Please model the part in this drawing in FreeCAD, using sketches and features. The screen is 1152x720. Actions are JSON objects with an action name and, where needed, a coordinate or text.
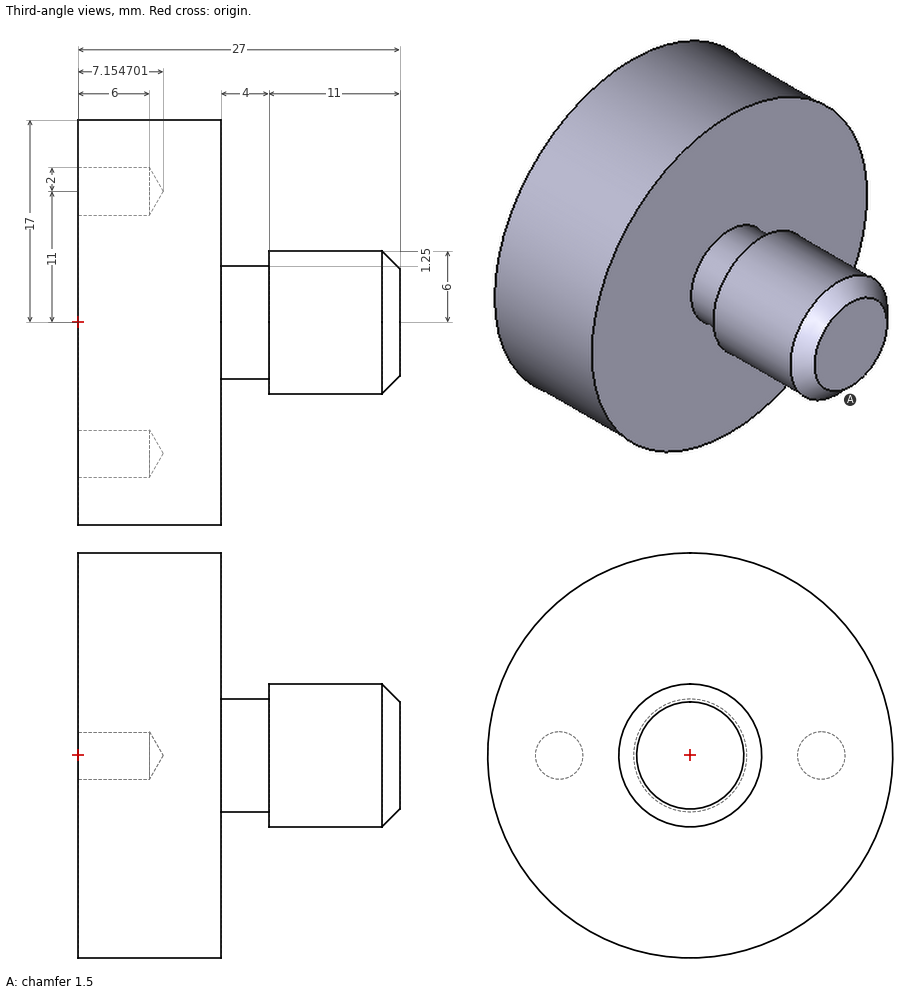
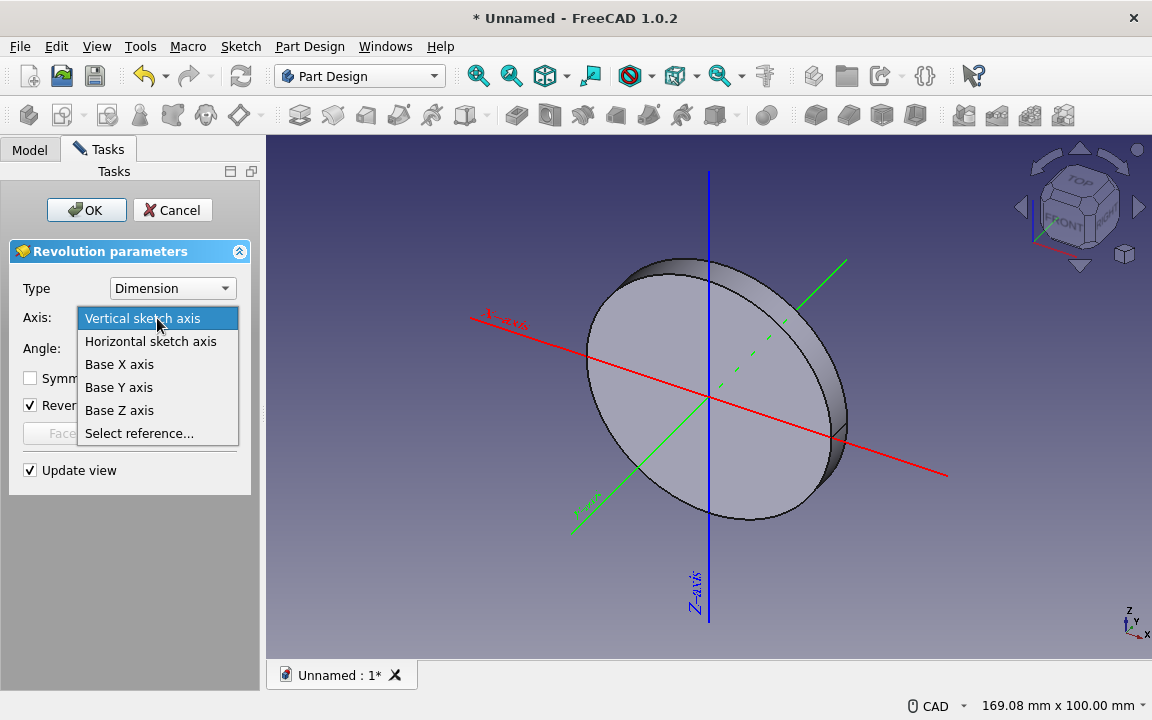
{"action": "left_click", "coordinate": [156, 342]}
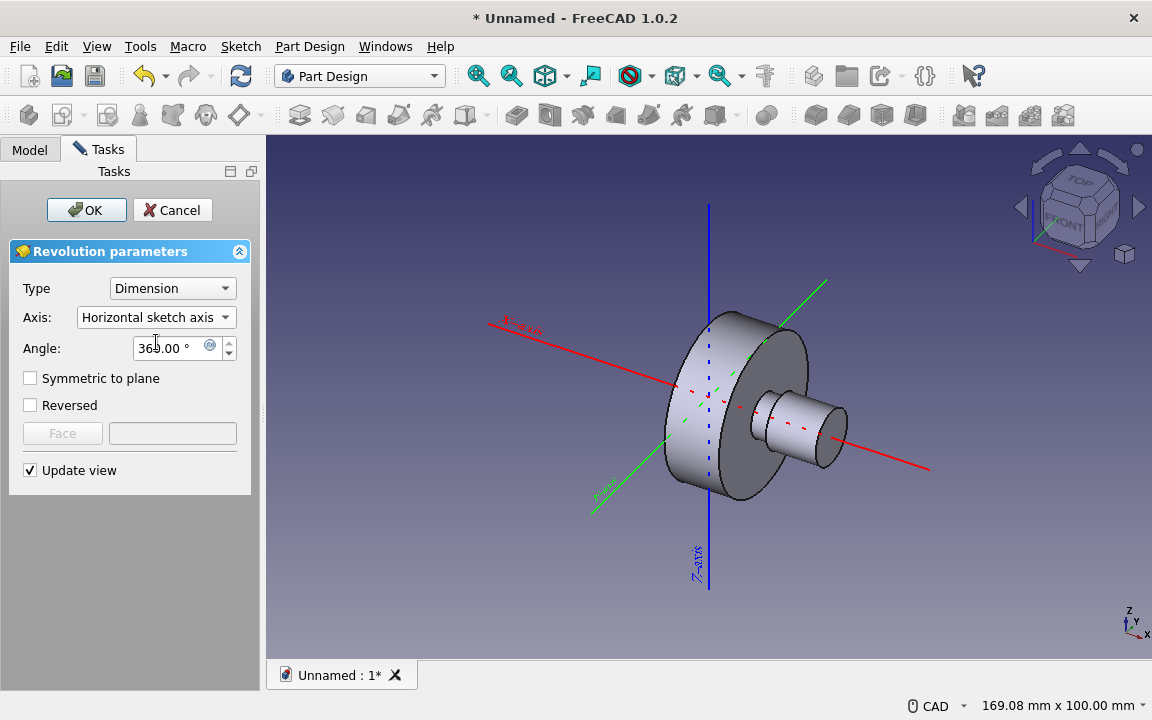
{"action": "left_click", "coordinate": [87, 210]}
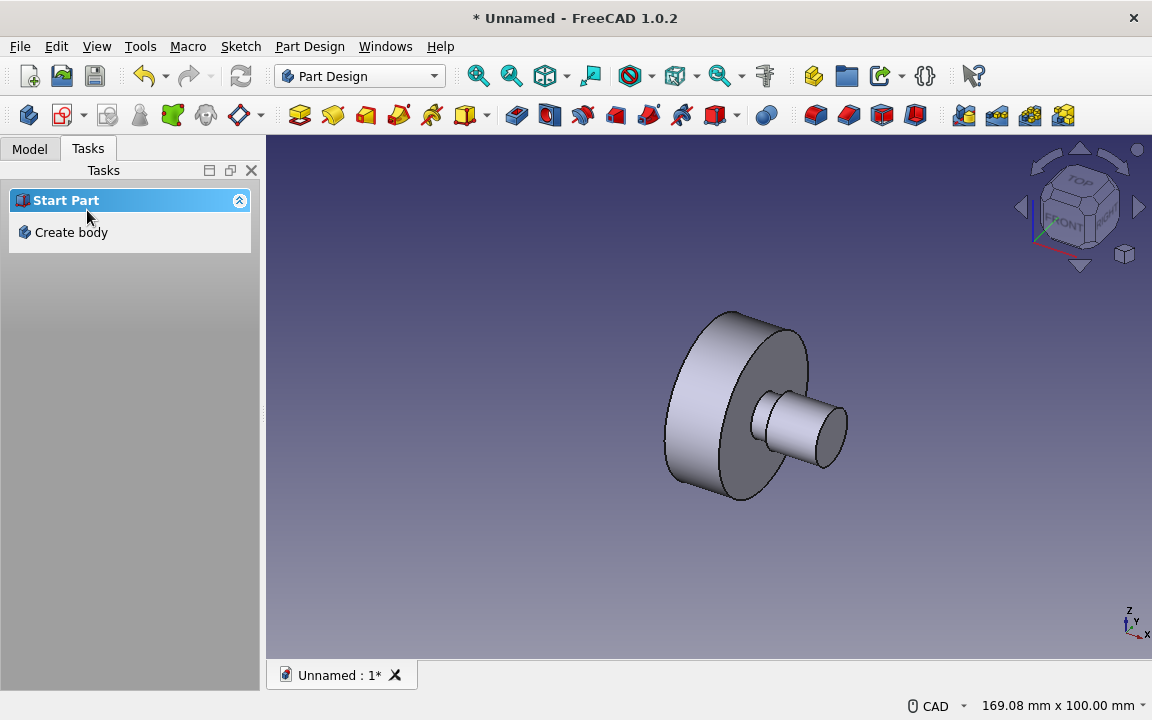
{"action": "left_click", "coordinate": [816, 452]}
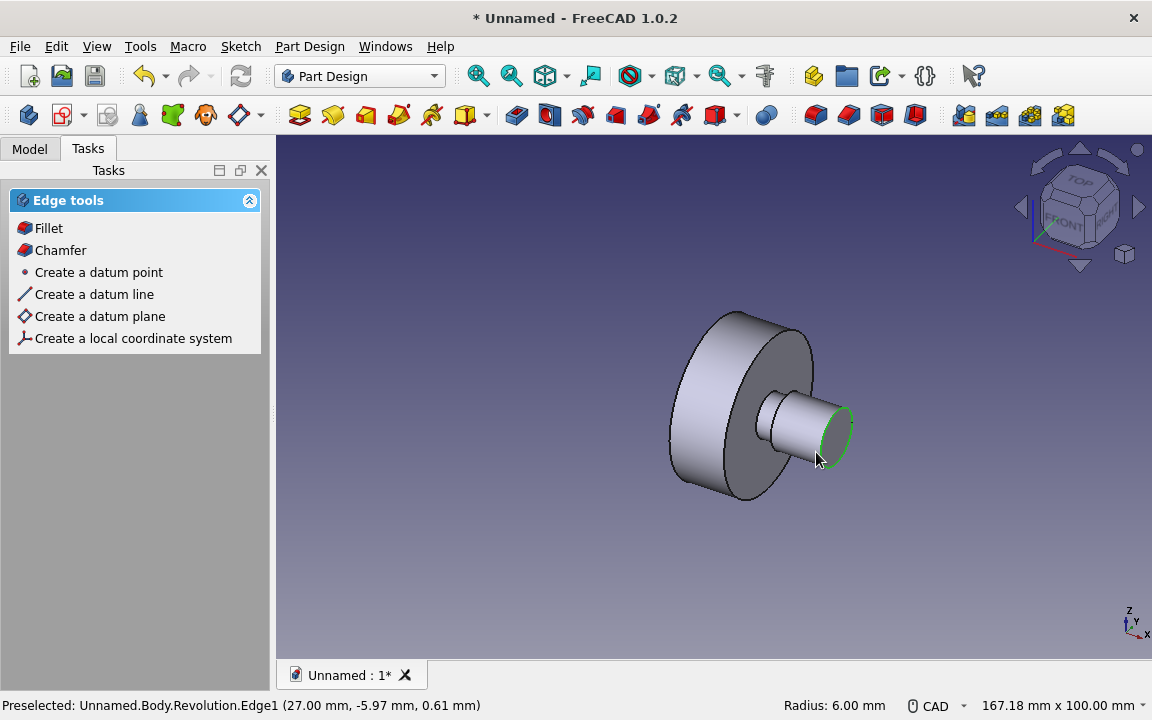
{"action": "left_click", "coordinate": [849, 116]}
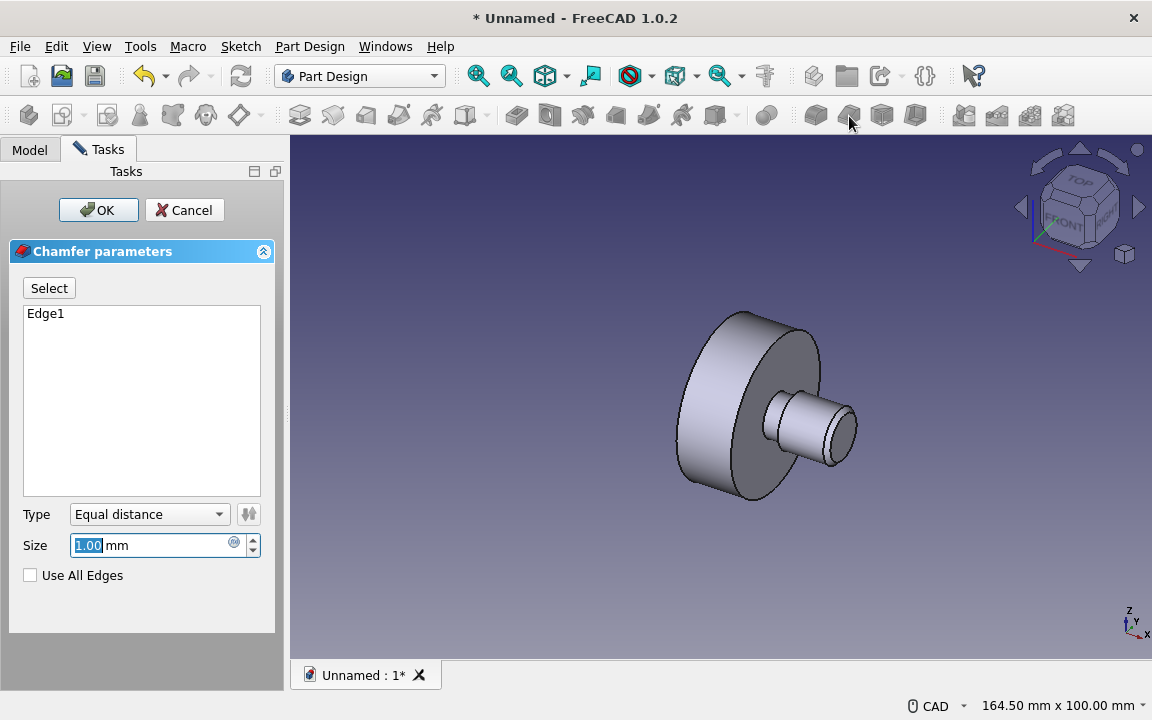
{"action": "type", "text": "1.5"}
{"action": "key", "text": "Tab"}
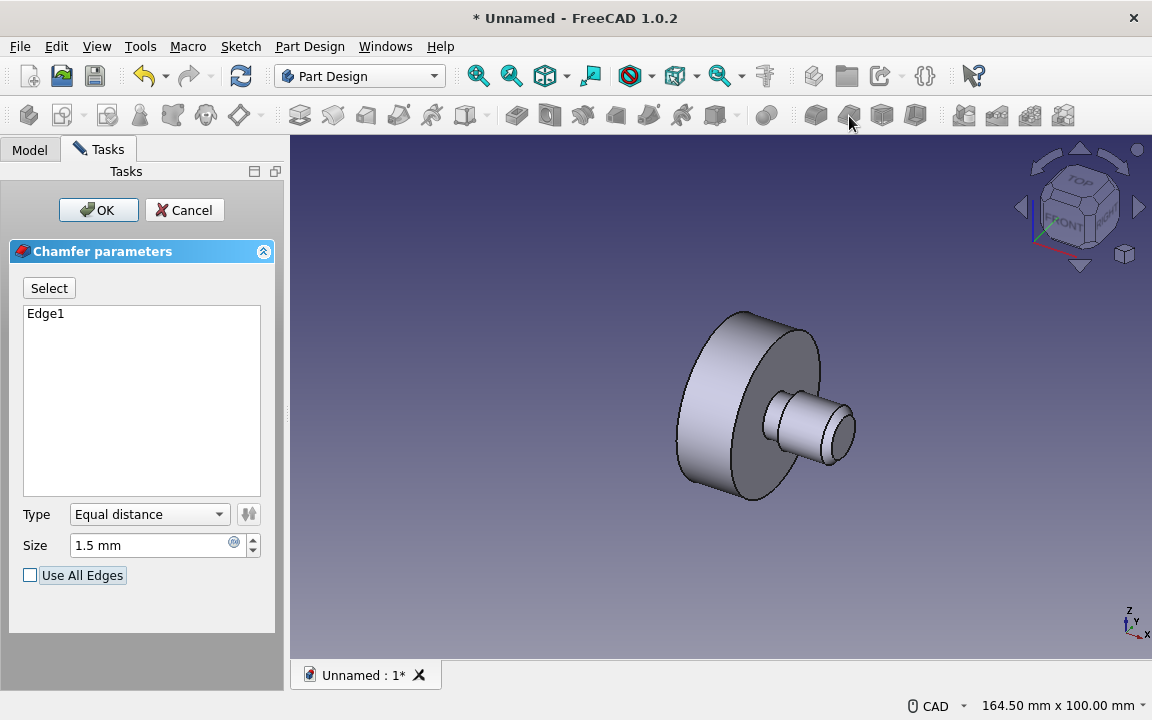
{"action": "left_click", "coordinate": [99, 210]}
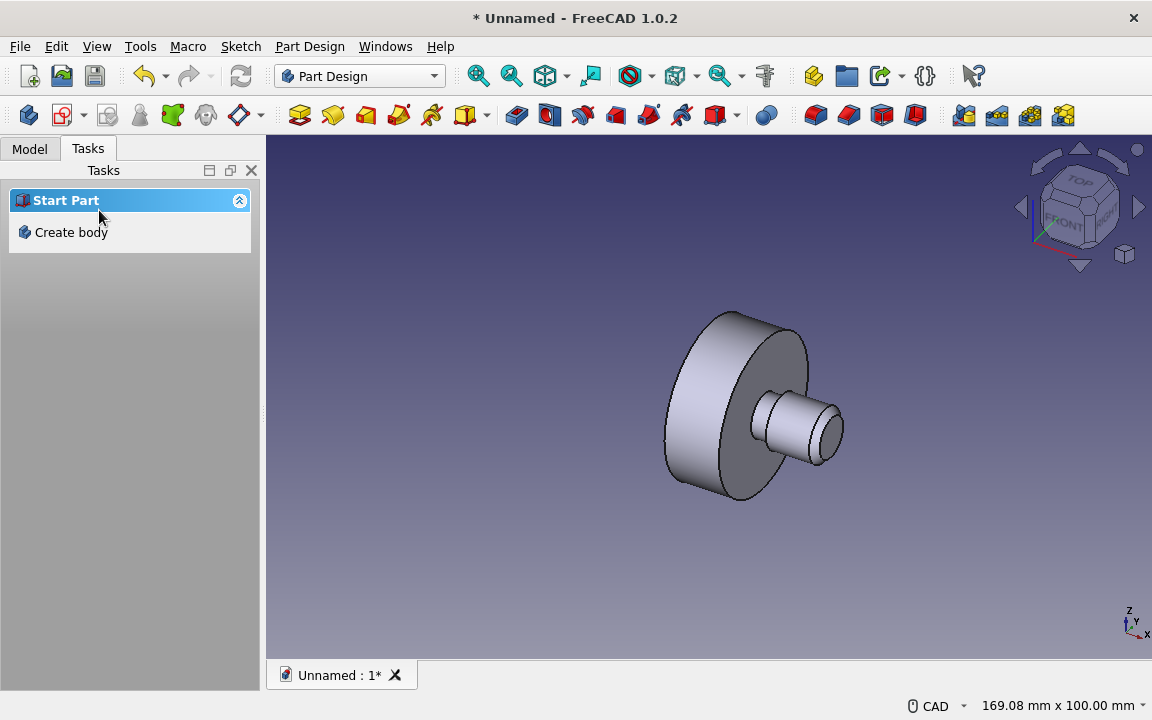
{"action": "left_click", "coordinate": [62, 116]}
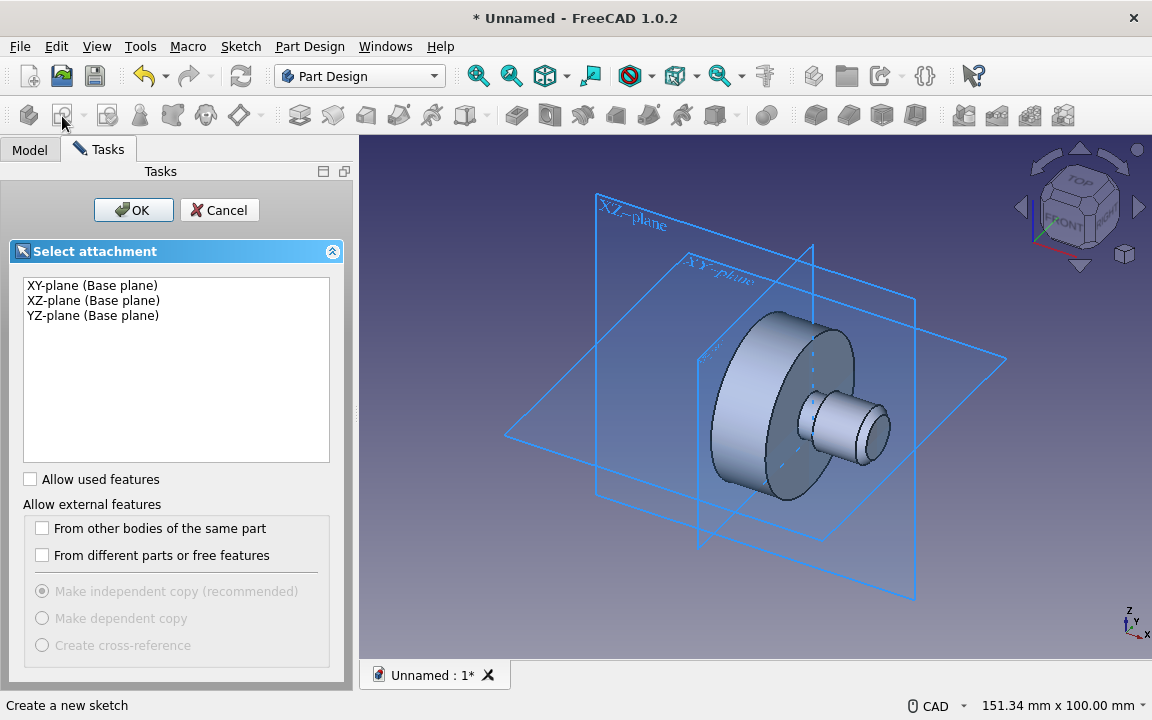
{"action": "left_click", "coordinate": [84, 286]}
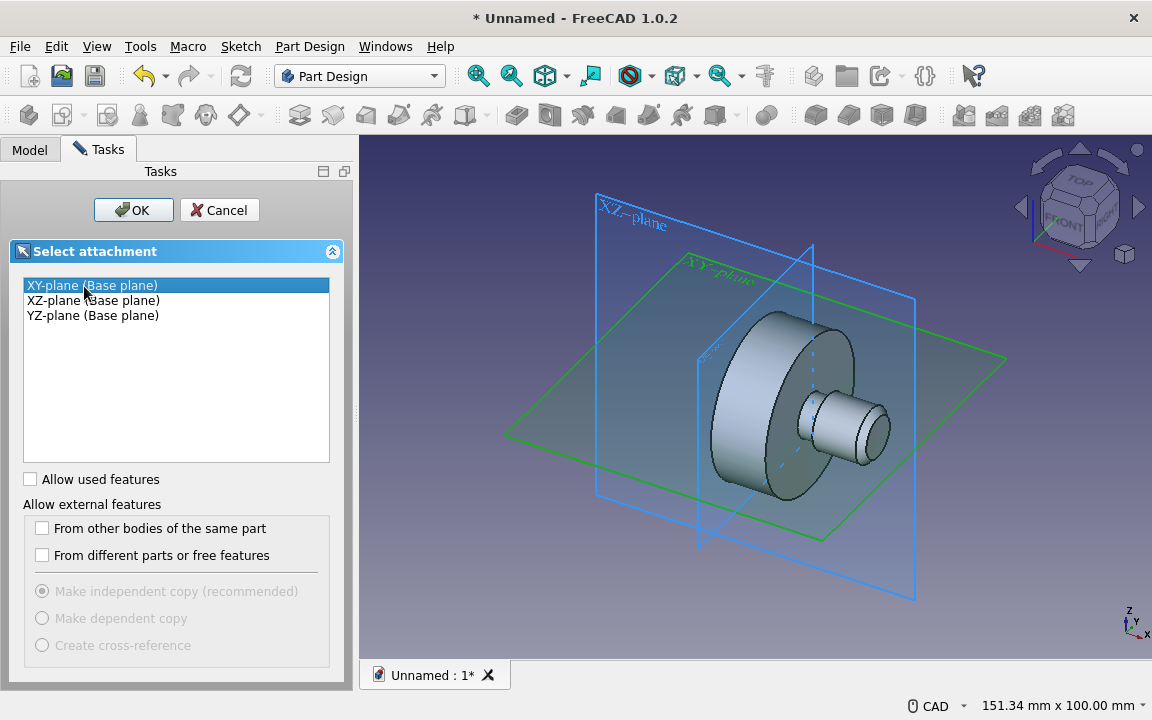
{"action": "left_click", "coordinate": [134, 210]}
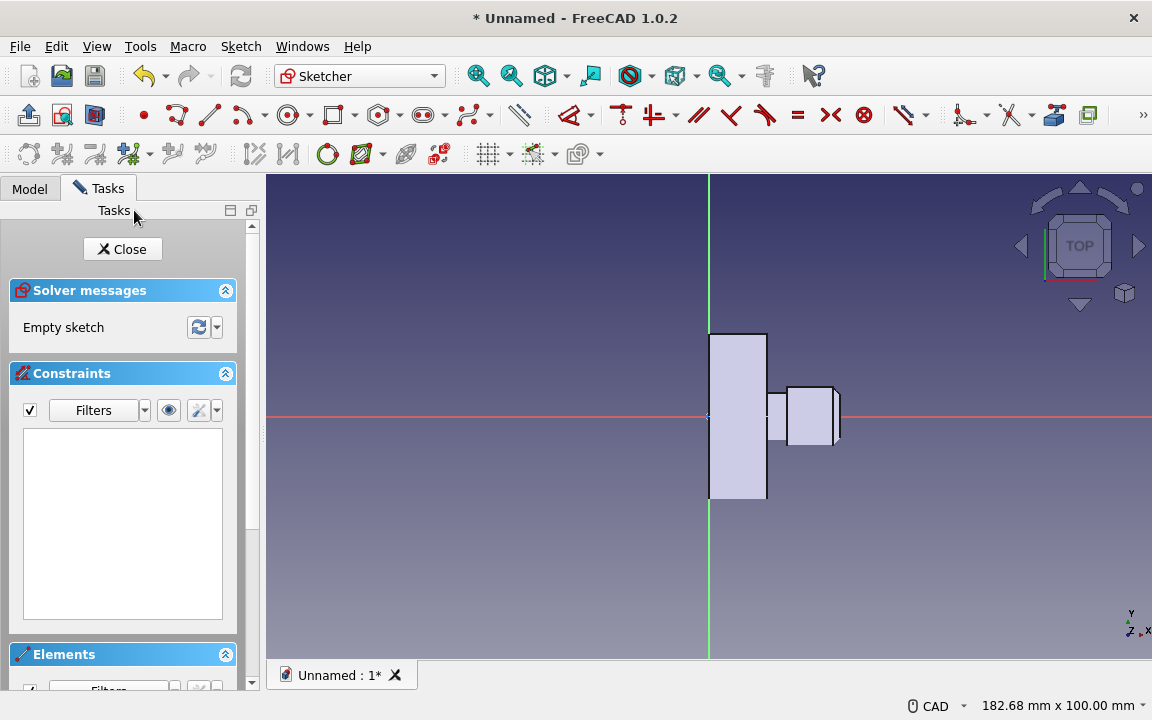
{"action": "key", "text": "q s"}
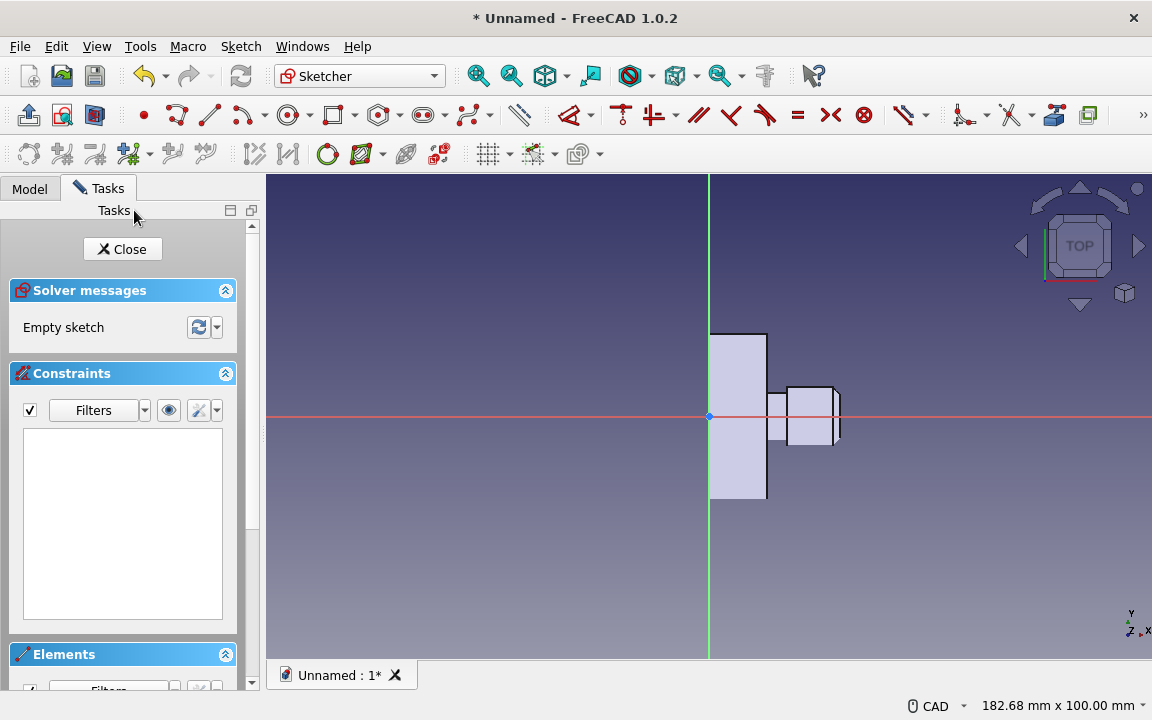
{"action": "scroll", "coordinate": [757, 377], "scroll_direction": "up", "scroll_amount": 8}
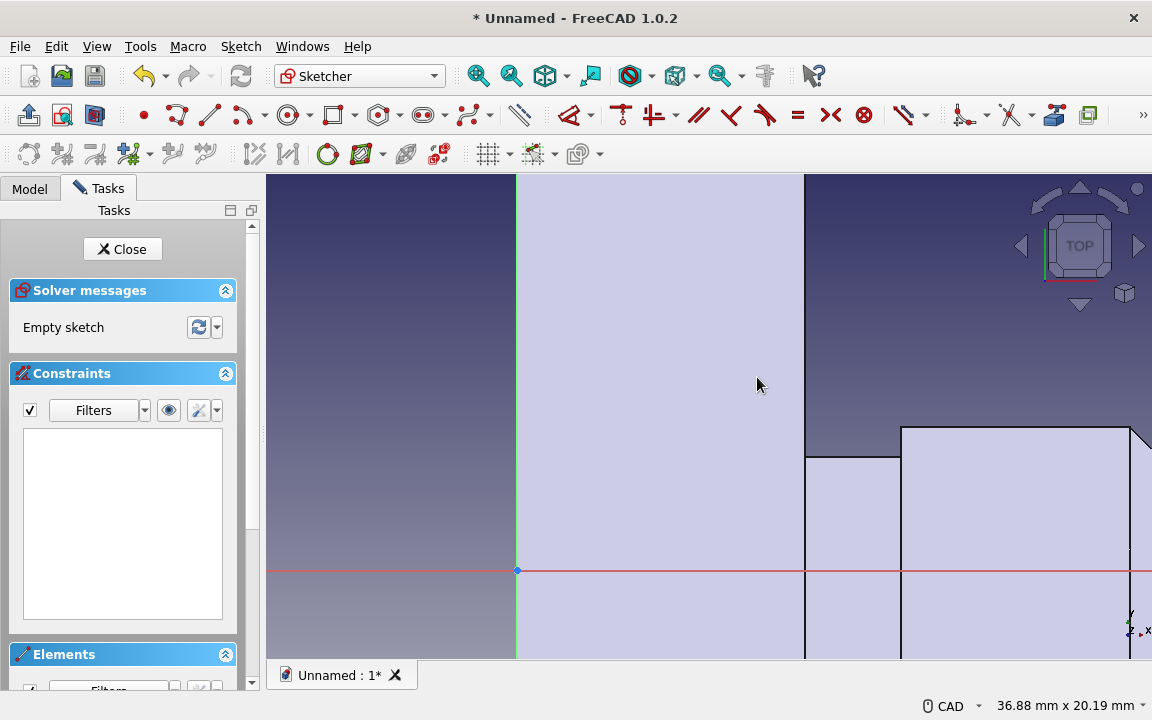
{"action": "left_click", "coordinate": [177, 116]}